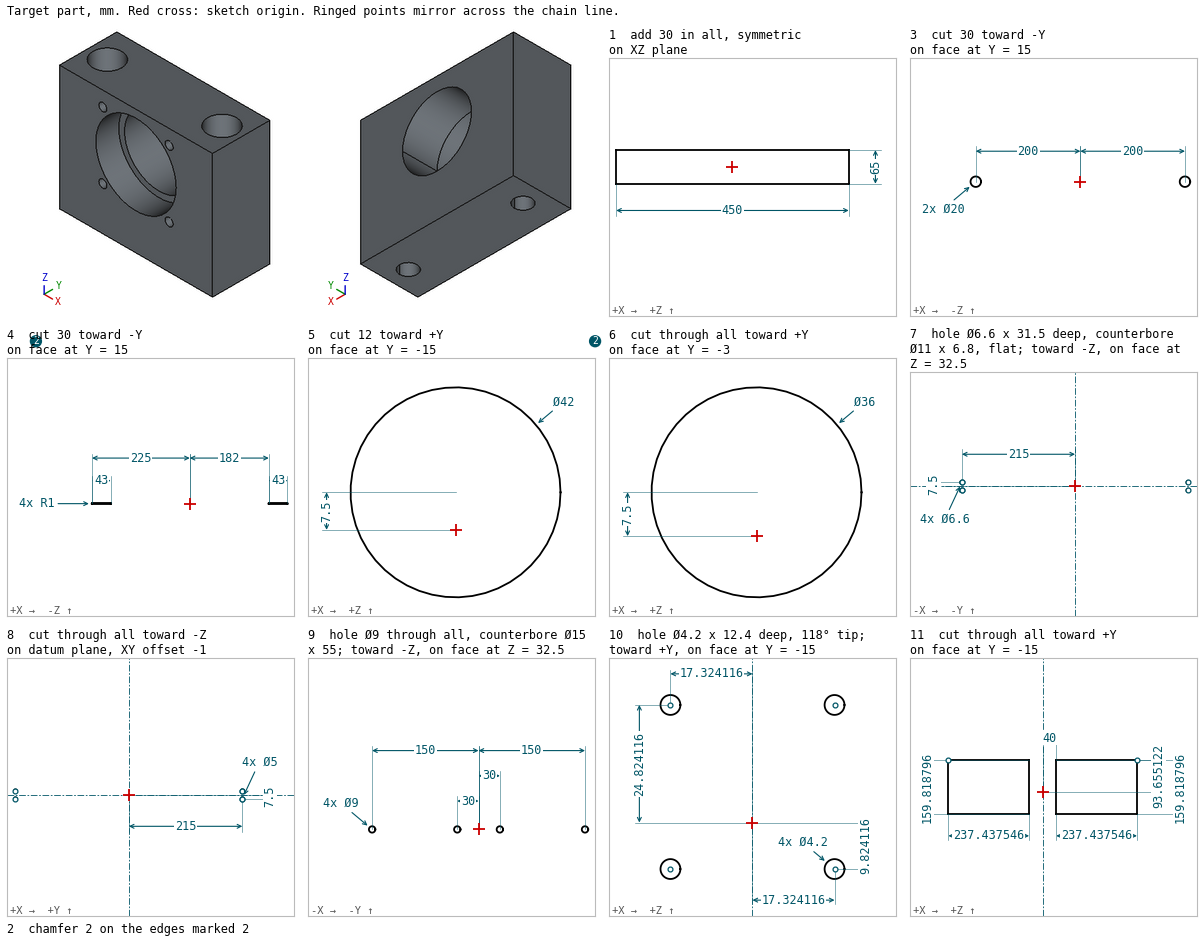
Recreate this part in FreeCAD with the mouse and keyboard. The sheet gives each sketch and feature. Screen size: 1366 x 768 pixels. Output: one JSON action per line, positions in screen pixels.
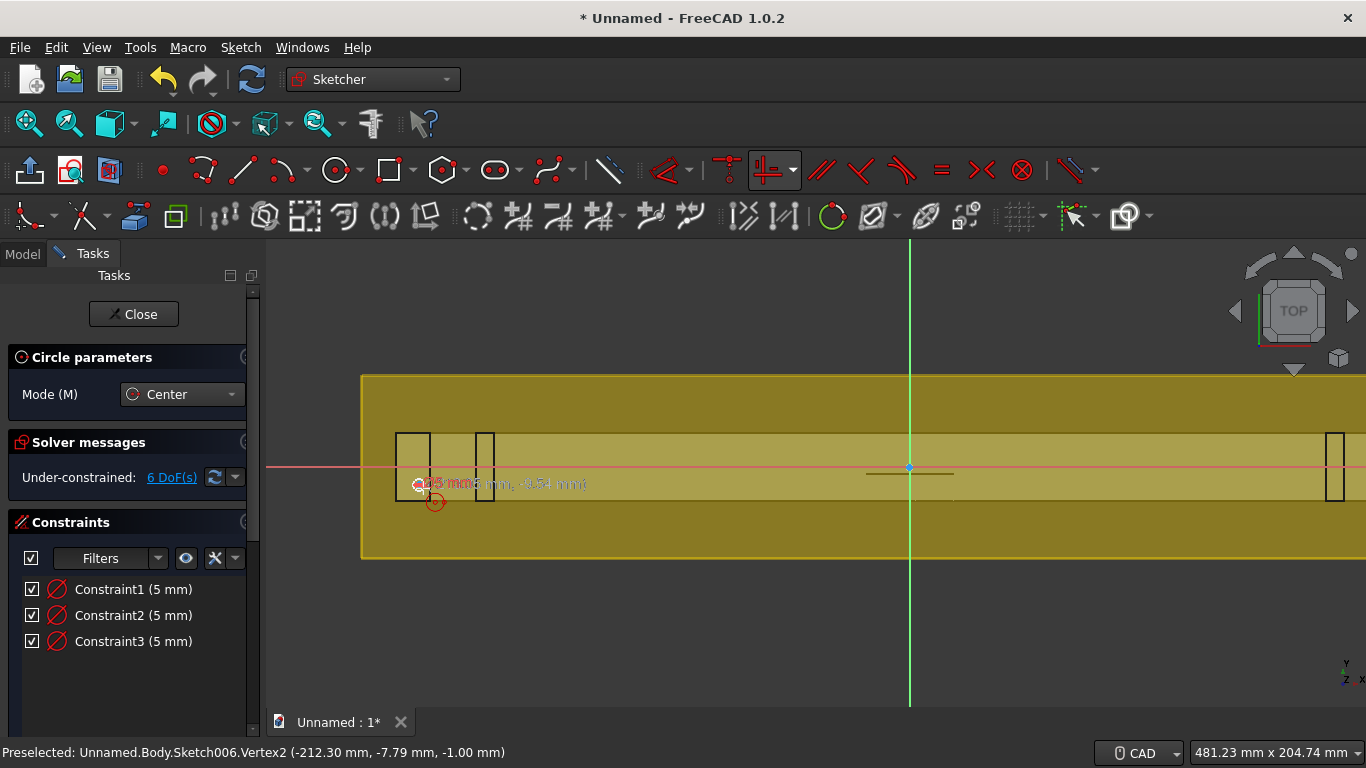
{"action": "scroll", "coordinate": [419, 450], "scroll_direction": "up", "scroll_amount": 7}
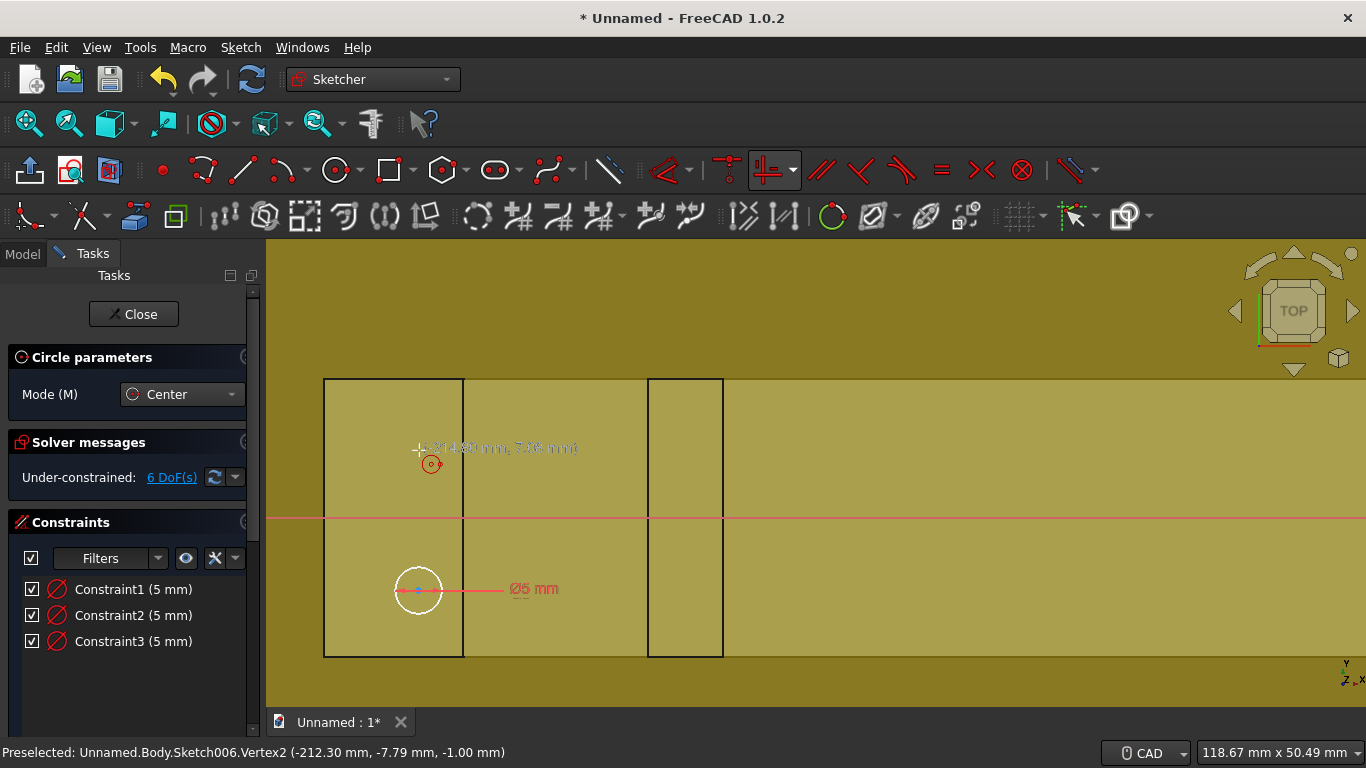
{"action": "scroll", "coordinate": [418, 464], "scroll_direction": "down", "scroll_amount": 9}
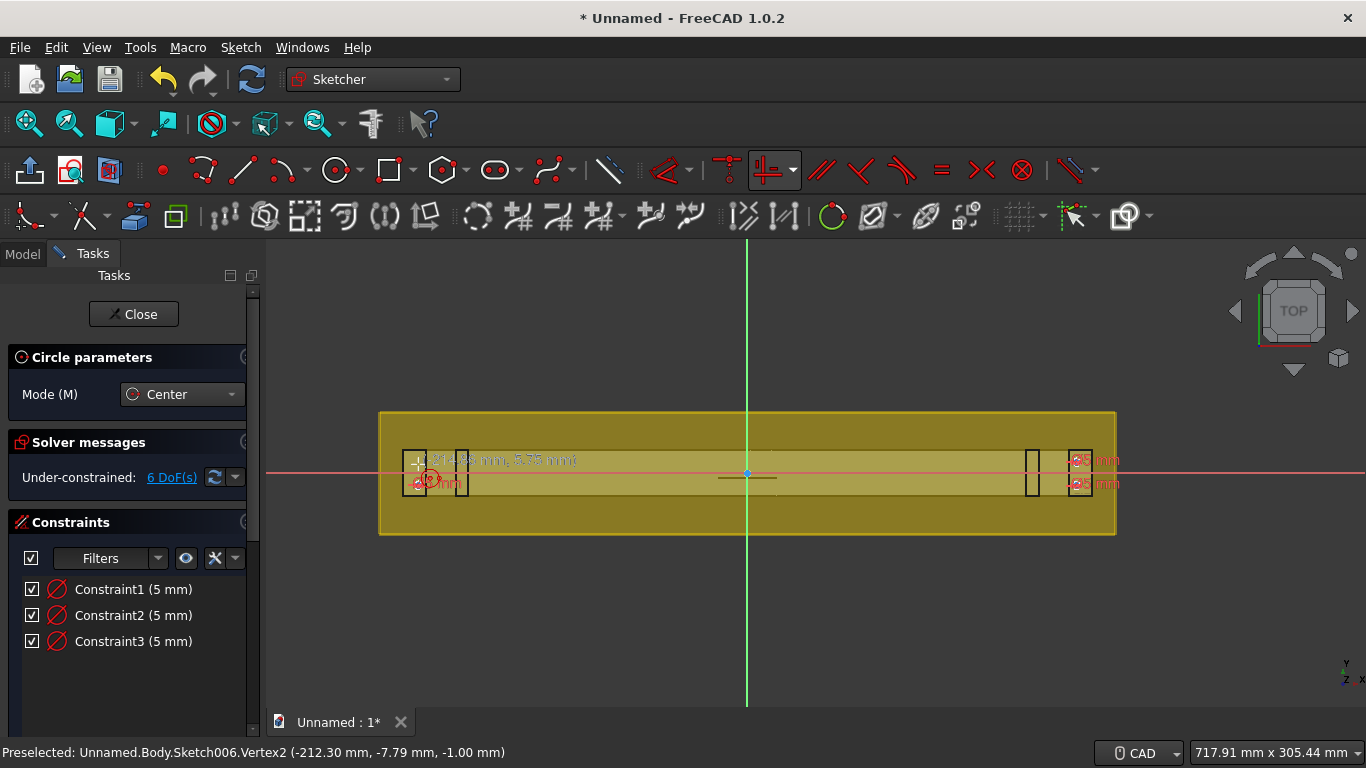
{"action": "scroll", "coordinate": [418, 462], "scroll_direction": "up", "scroll_amount": 2}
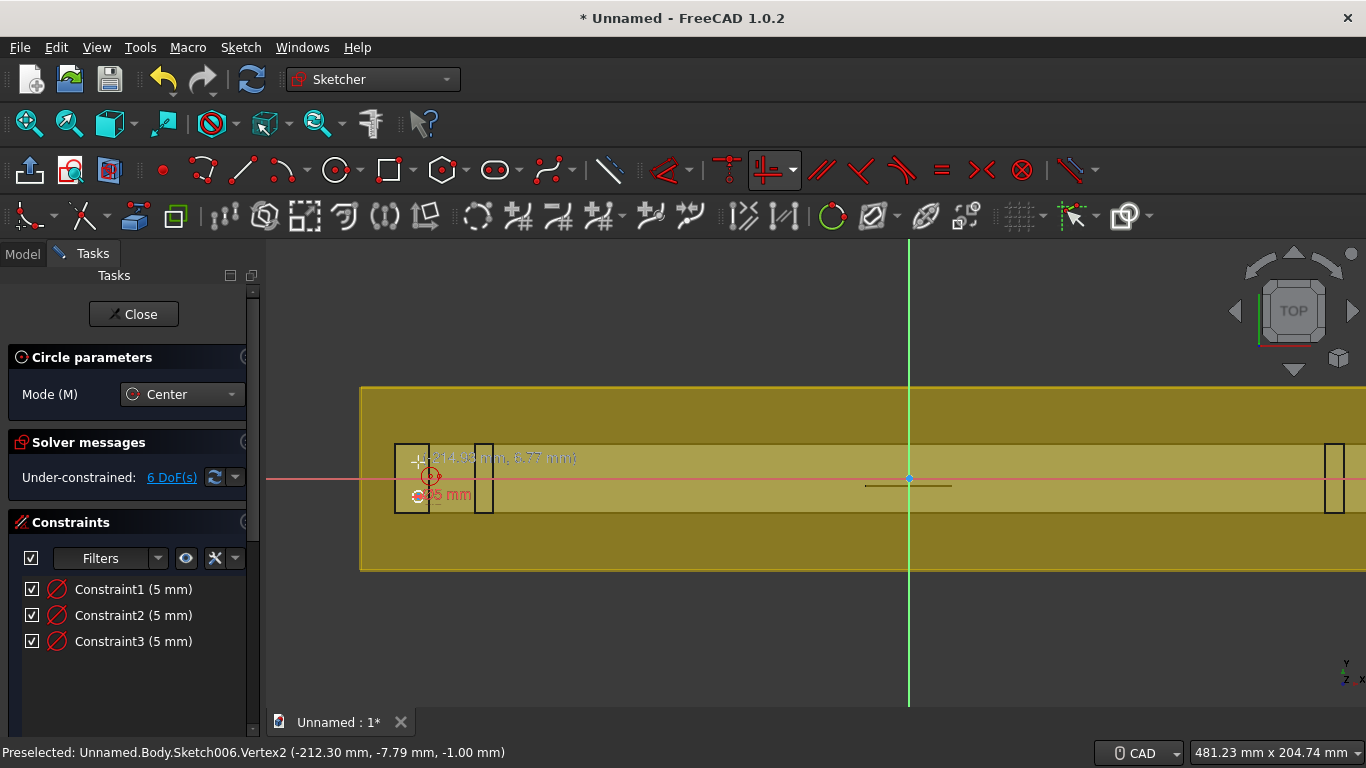
{"action": "left_click", "coordinate": [418, 462]}
{"action": "mouse_move", "coordinate": [422, 458]}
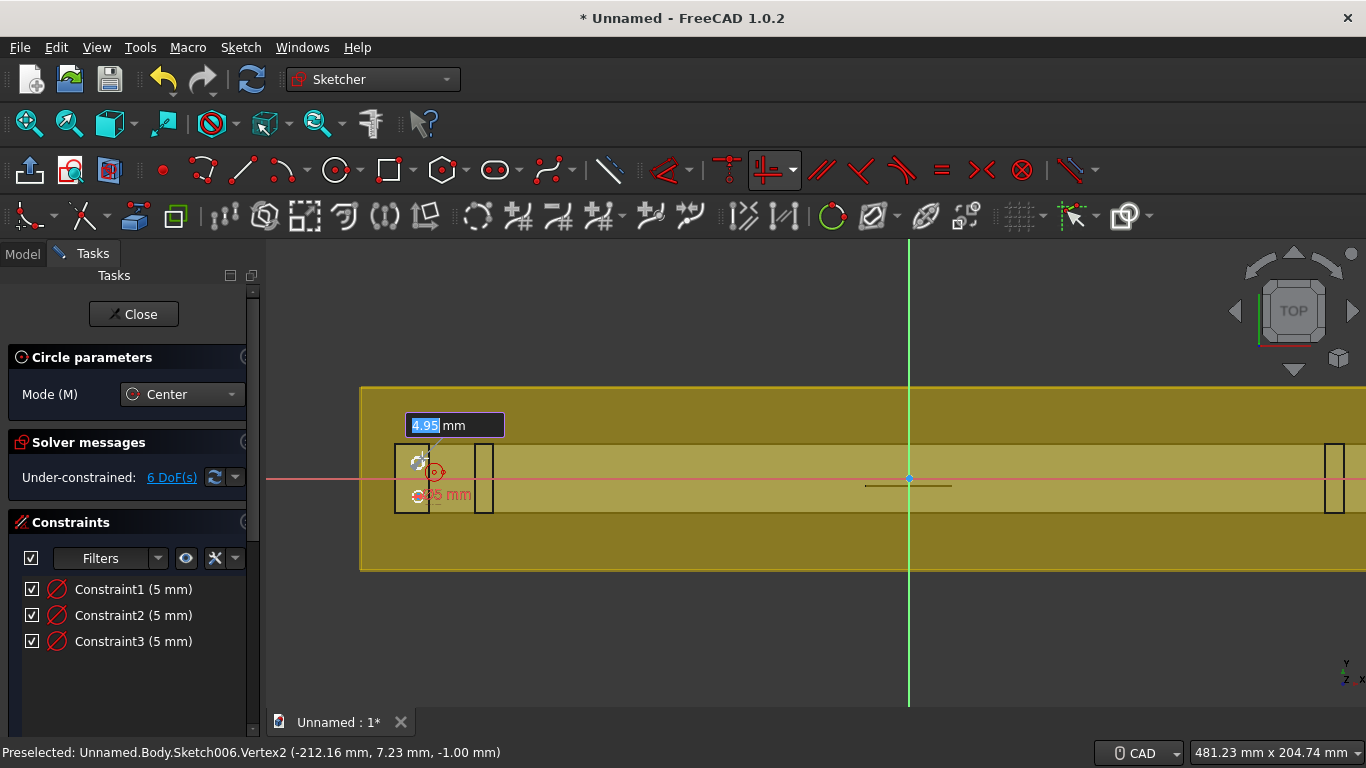
{"action": "type", "text": "5"}
{"action": "key", "text": "Return"}
{"action": "key", "text": "Escape"}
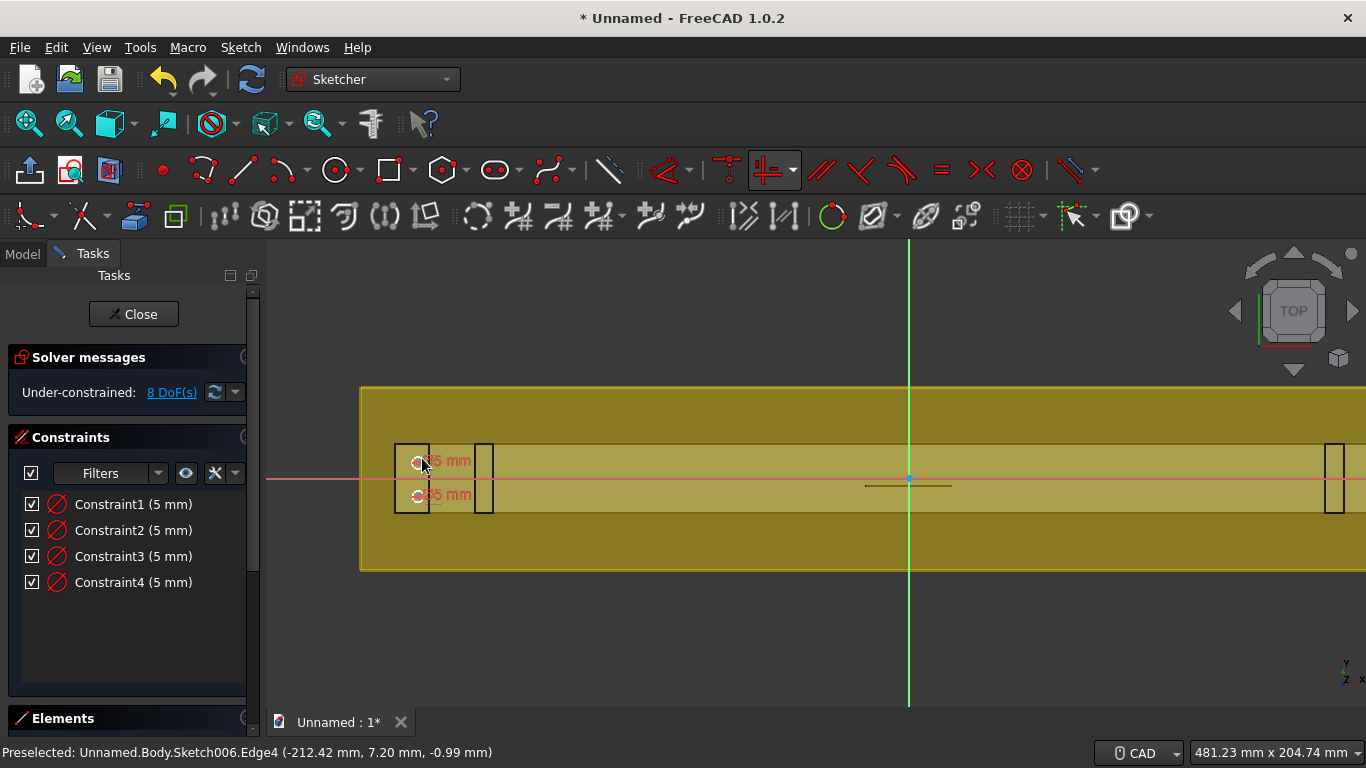
{"action": "scroll", "coordinate": [419, 461], "scroll_direction": "down", "scroll_amount": 2}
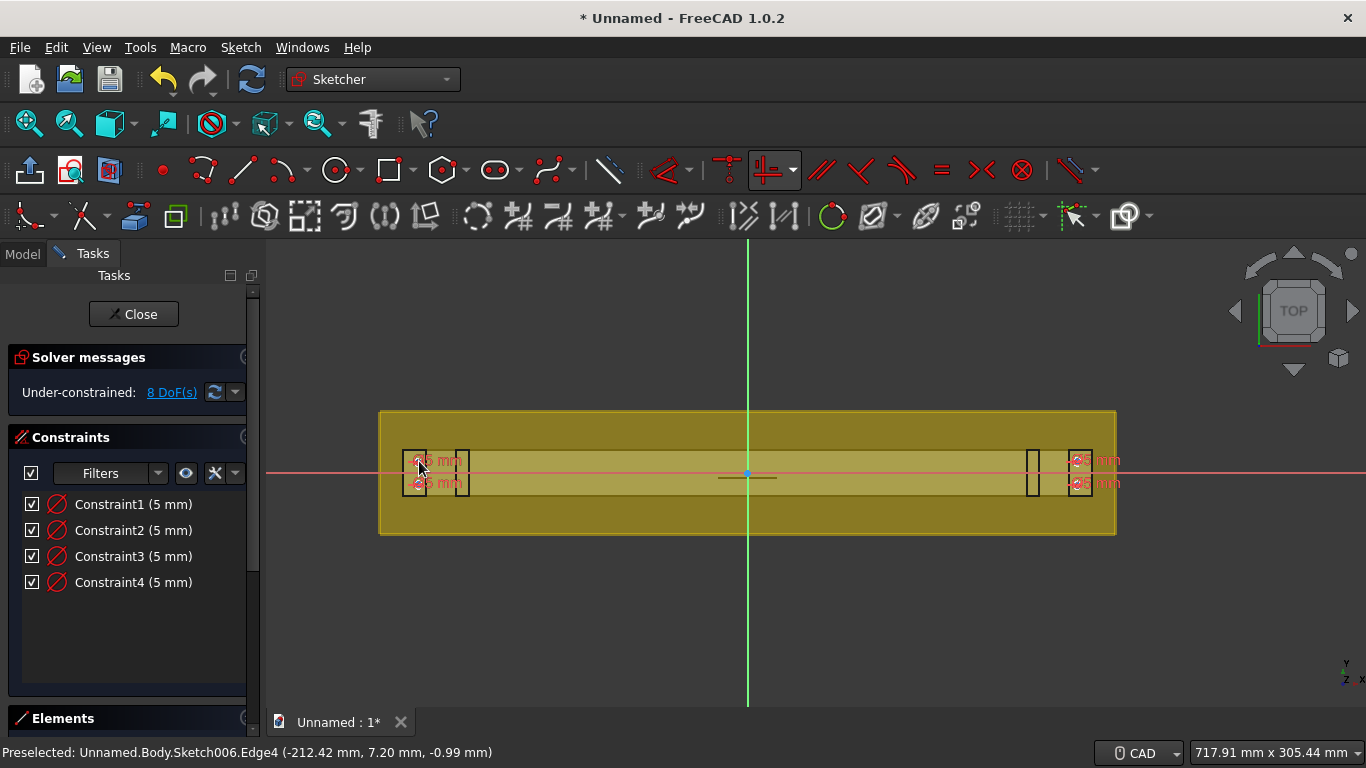
{"action": "left_click", "coordinate": [1077, 485]}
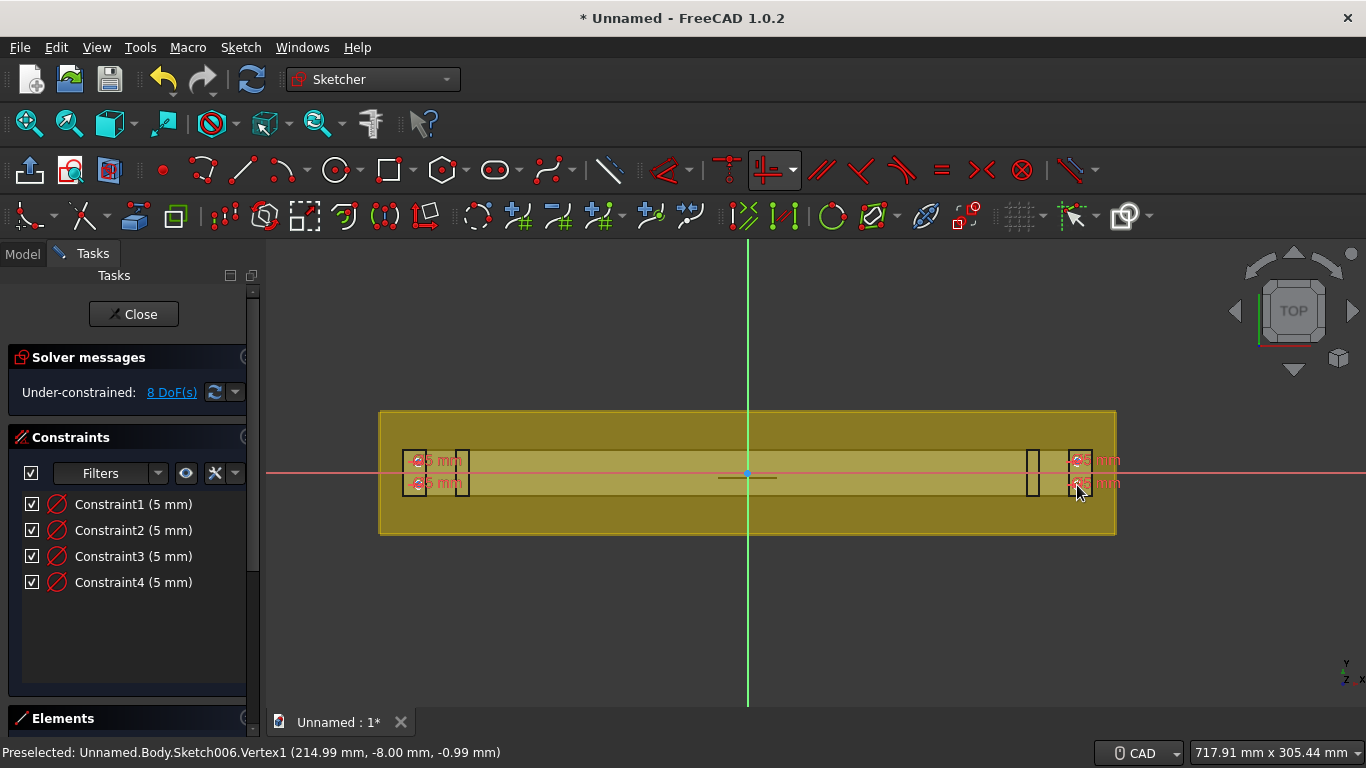
{"action": "left_click", "coordinate": [1077, 462]}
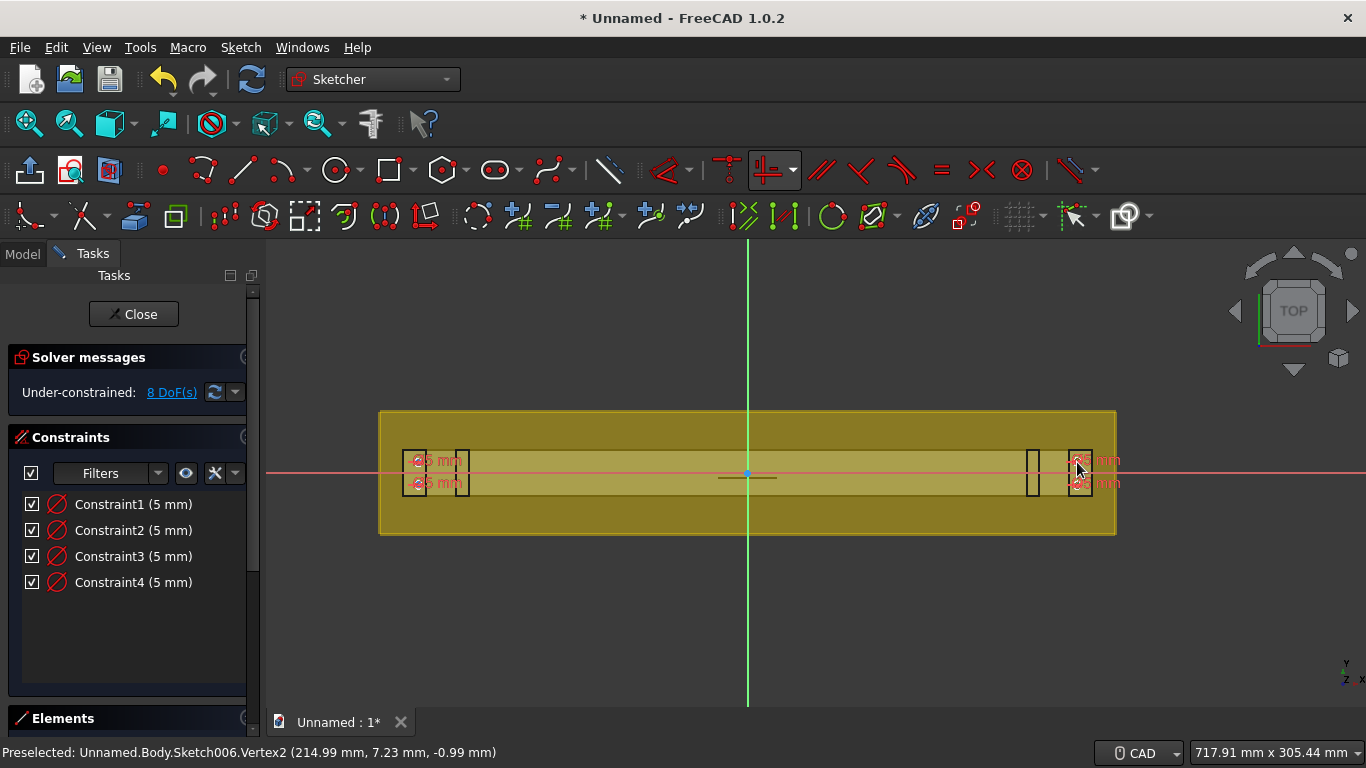
{"action": "left_click", "coordinate": [359, 473]}